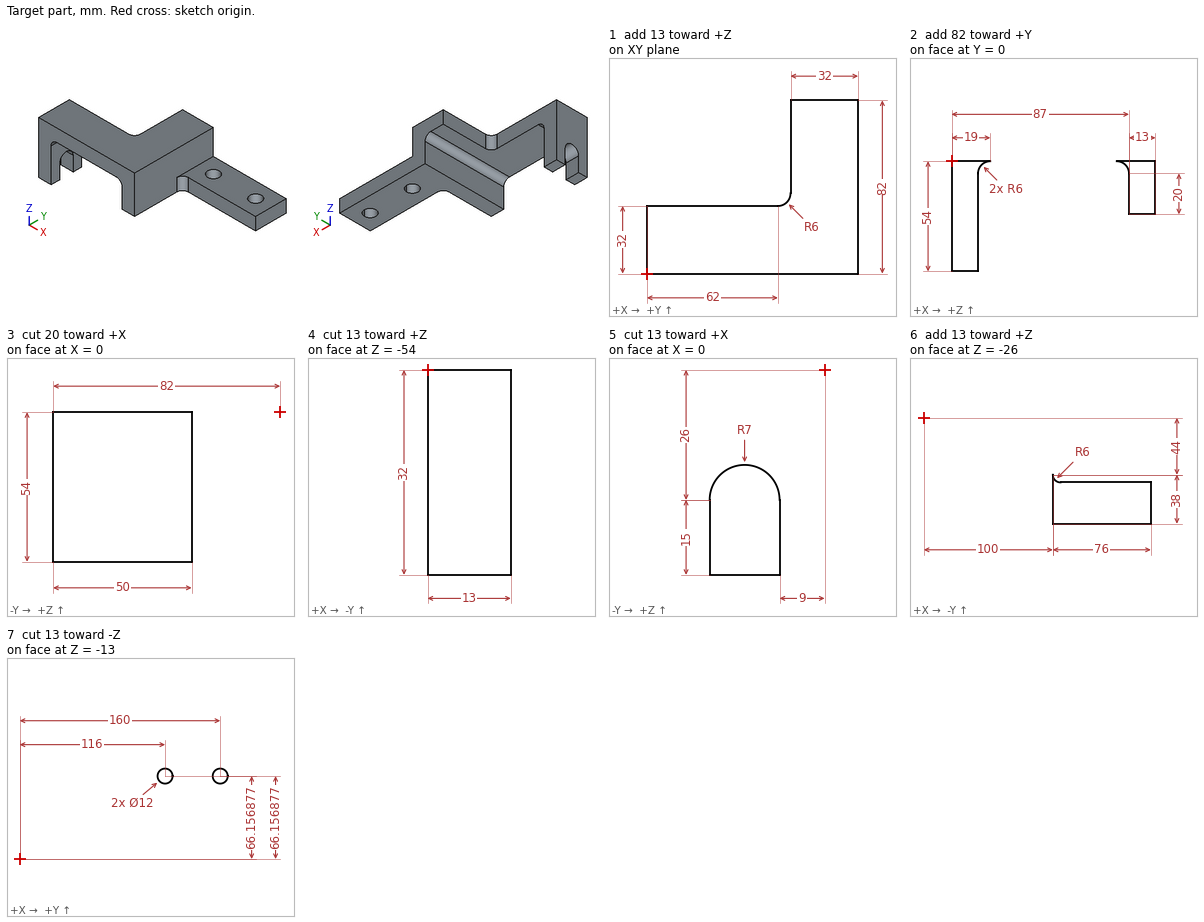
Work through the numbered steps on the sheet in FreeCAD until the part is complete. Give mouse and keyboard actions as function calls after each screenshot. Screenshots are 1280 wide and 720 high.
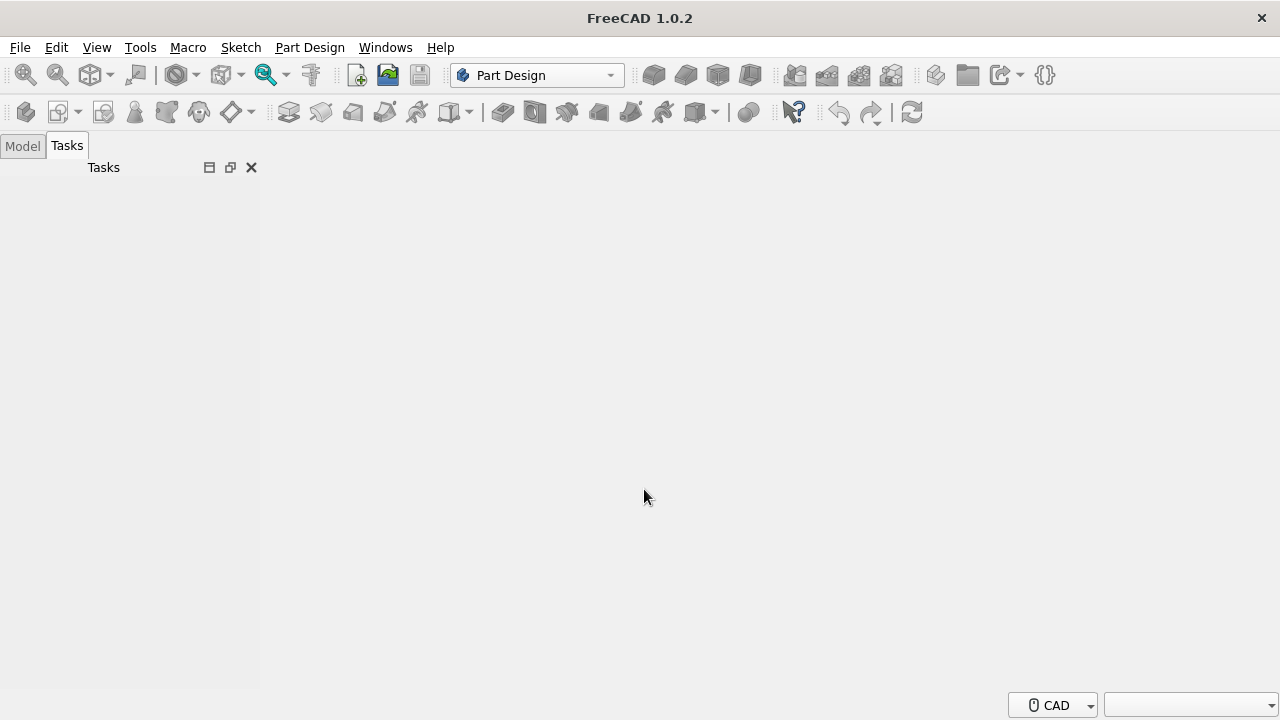
click(356, 76)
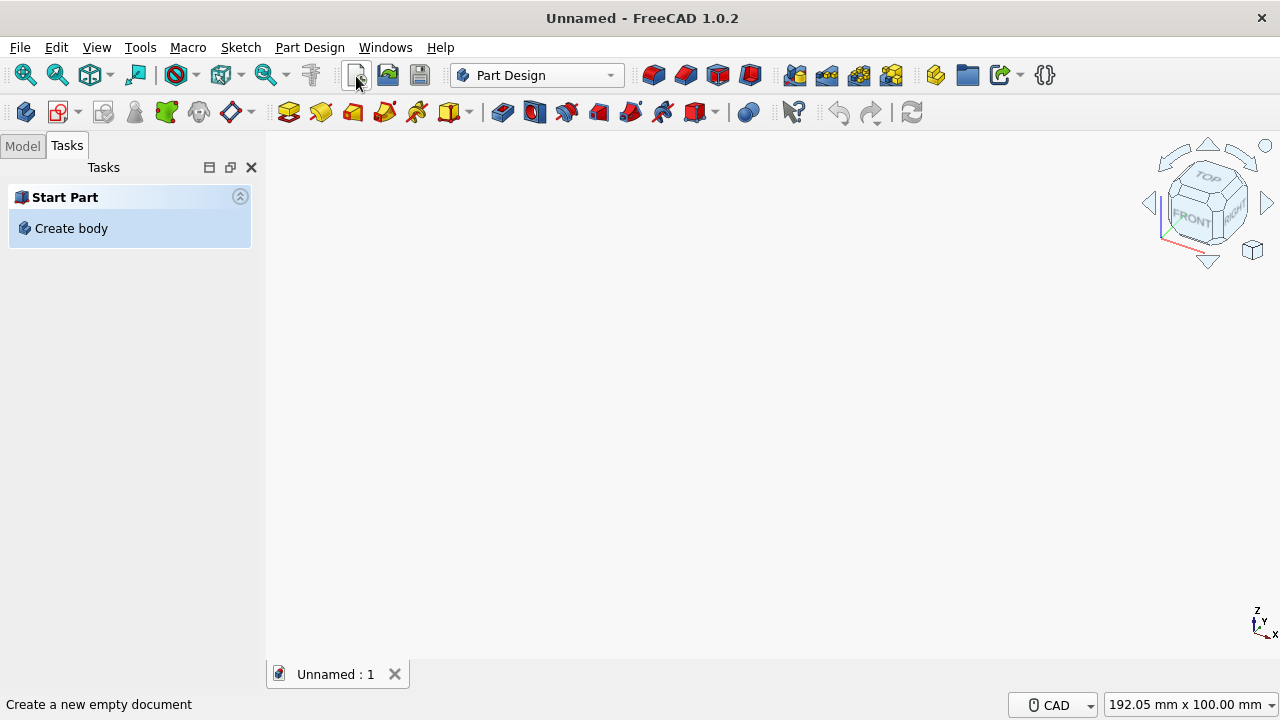
click(58, 112)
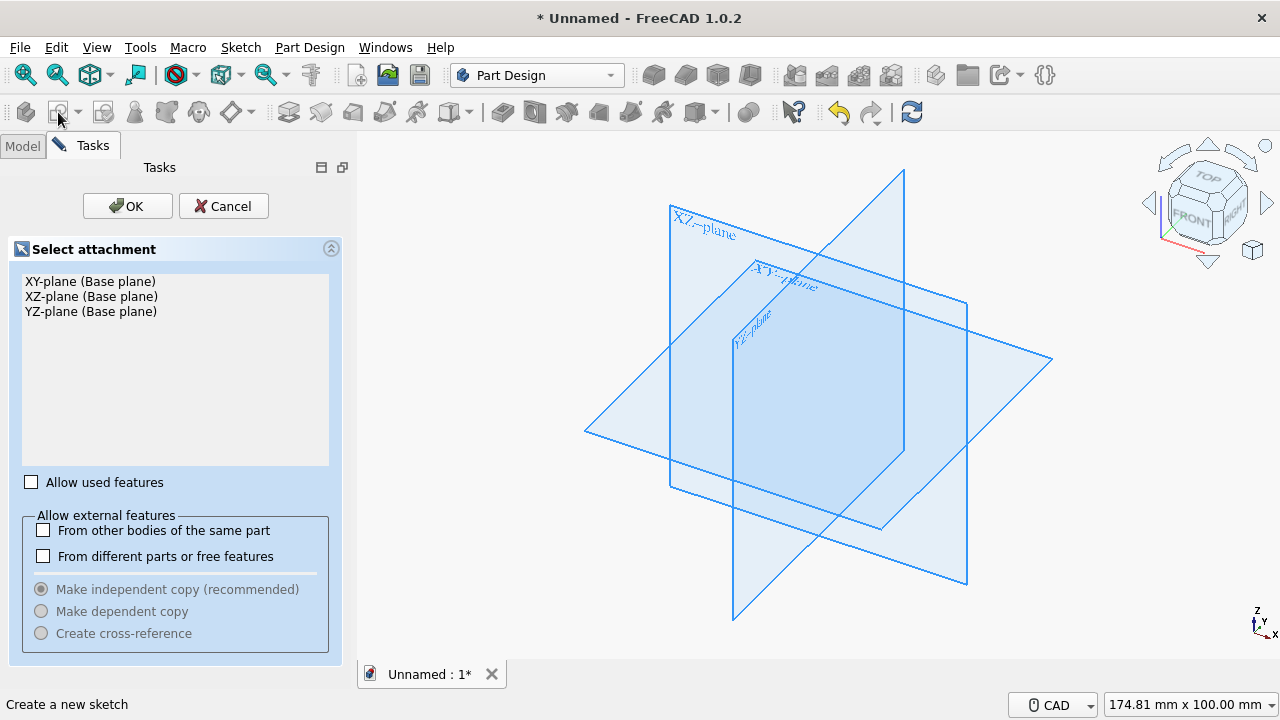
click(82, 282)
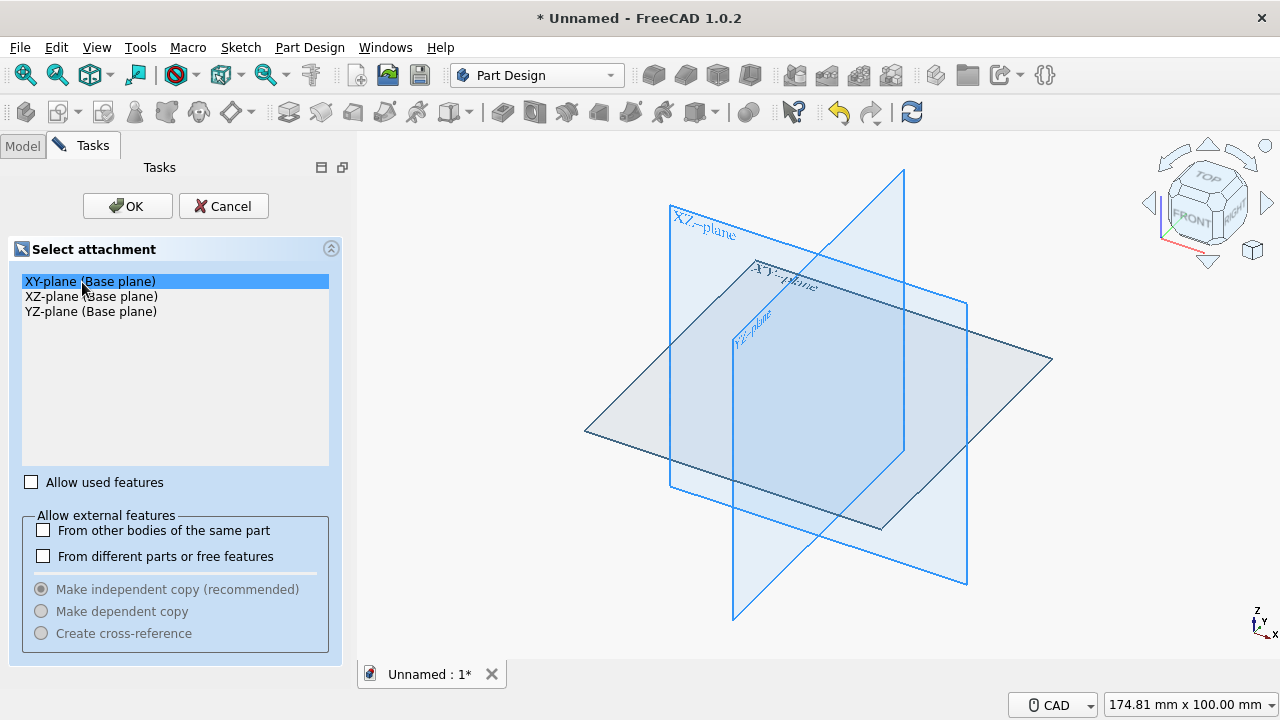
click(128, 206)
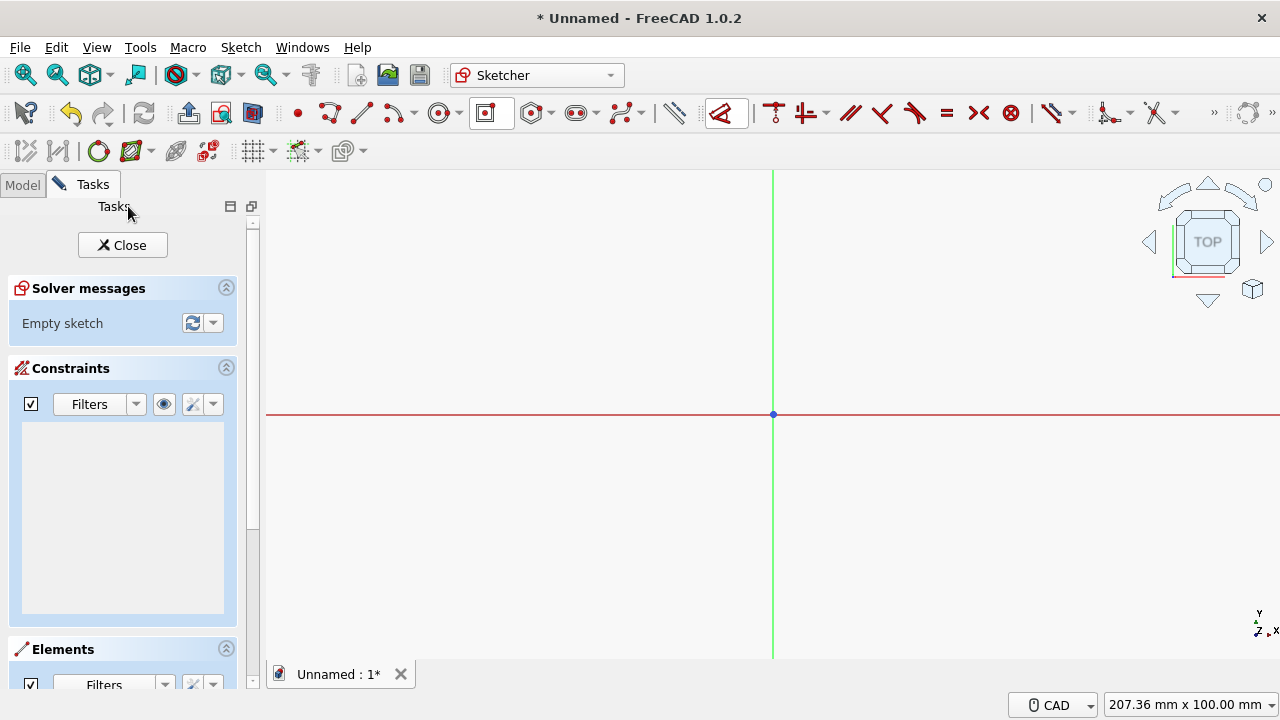
scroll(324, 631, down, 3)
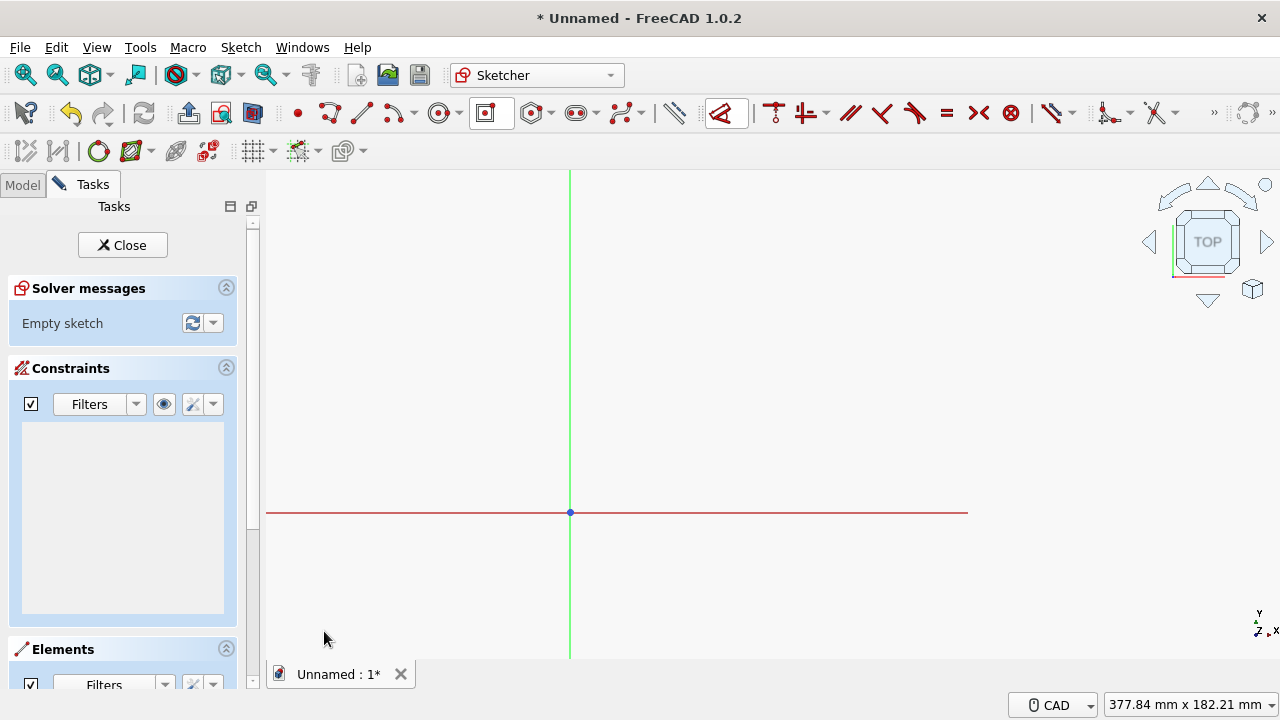
scroll(705, 378, up, 2)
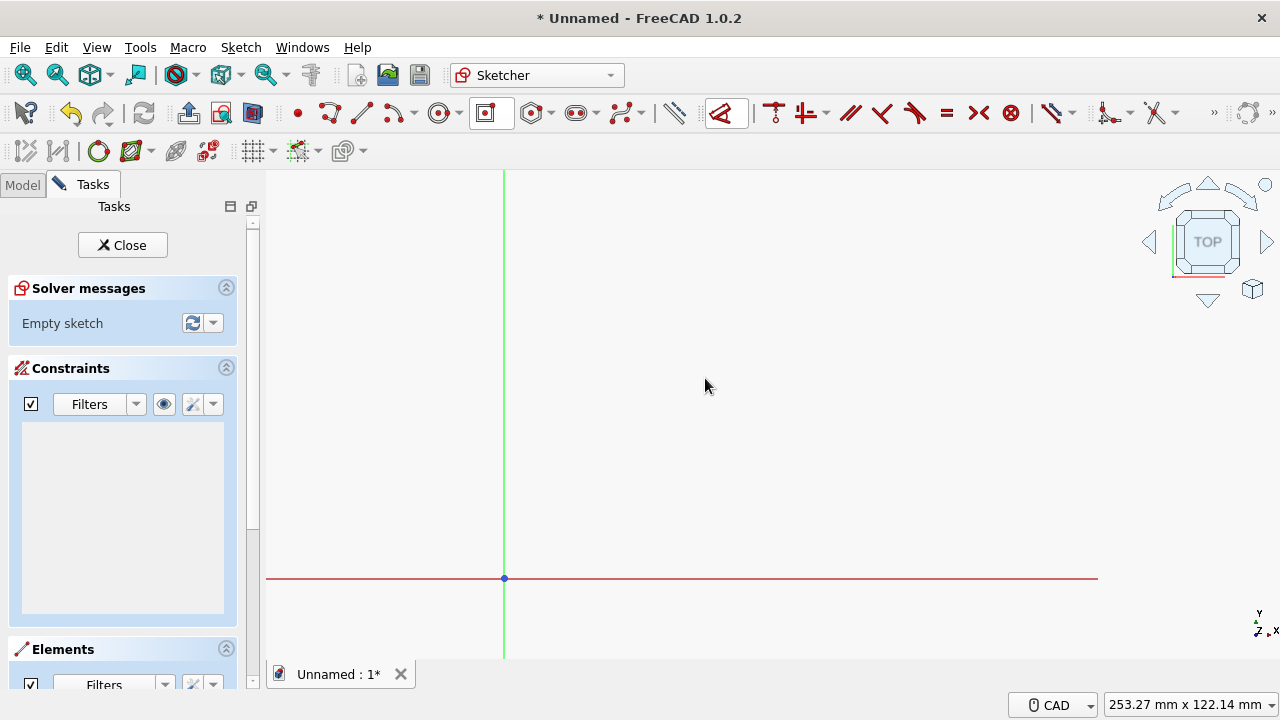
click(330, 114)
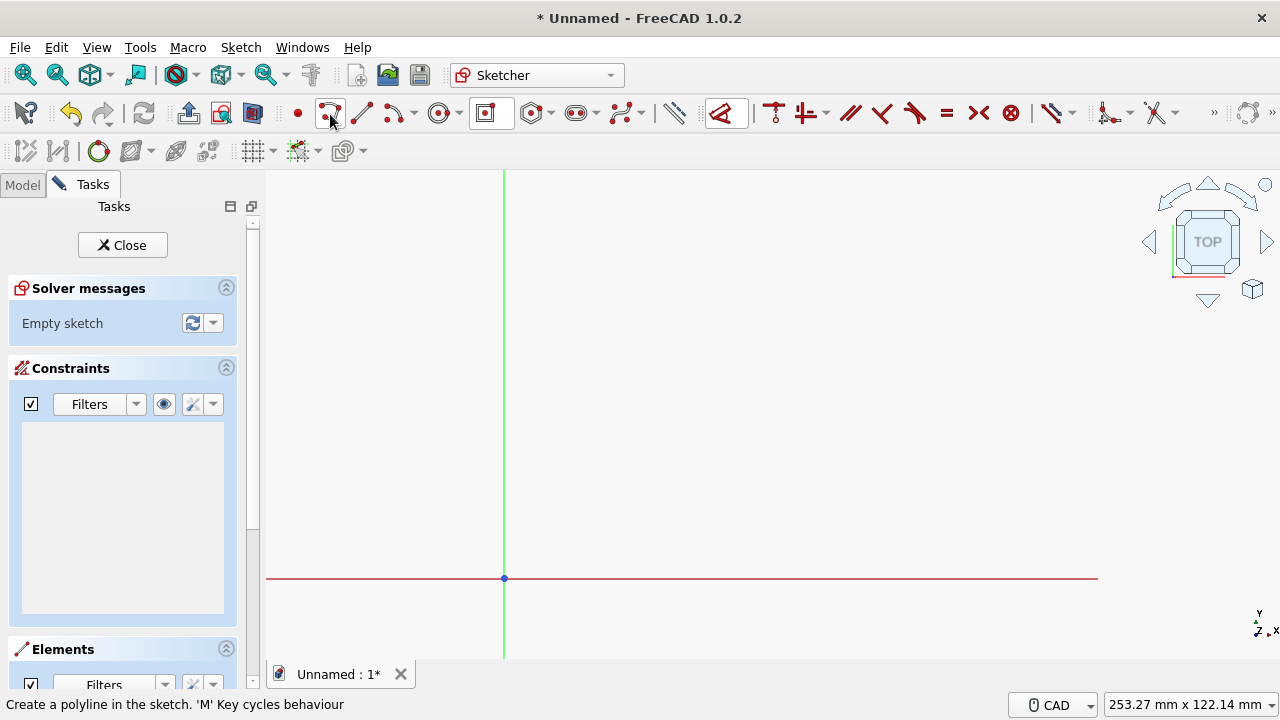
click(752, 450)
click(504, 450)
click(504, 579)
click(904, 570)
click(904, 250)
click(776, 250)
click(776, 426)
right_click(776, 426)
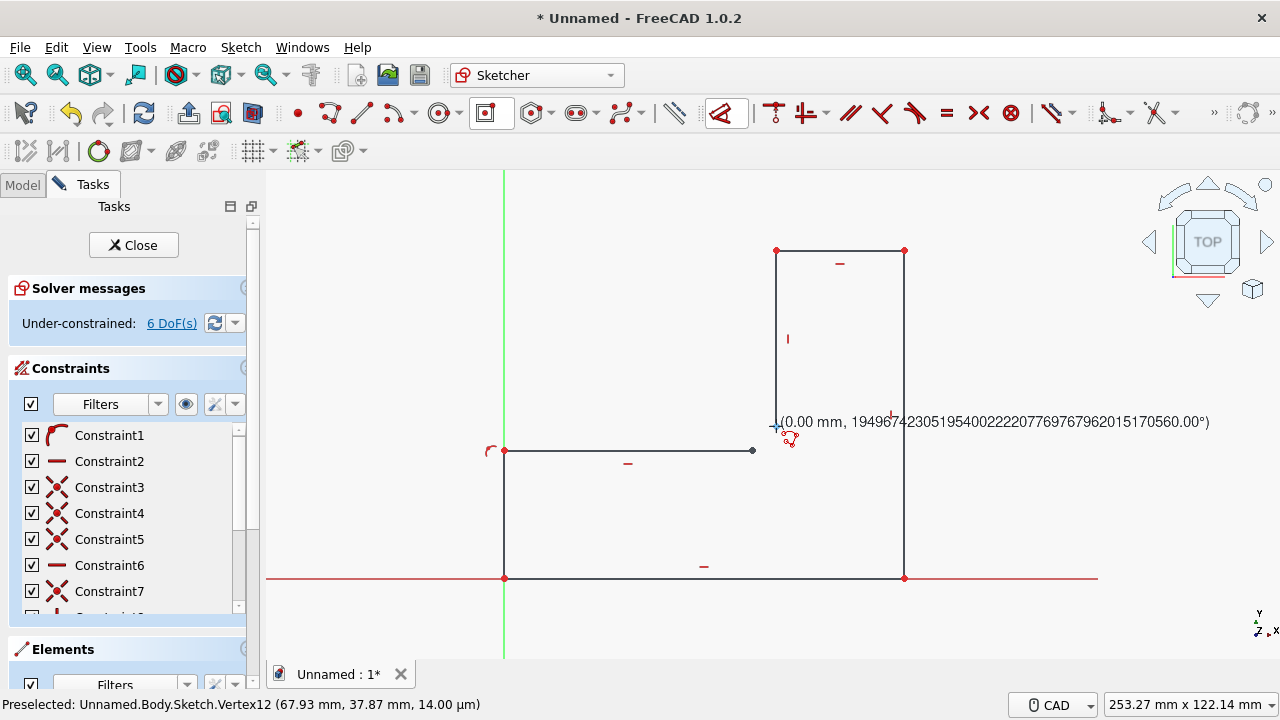
click(416, 114)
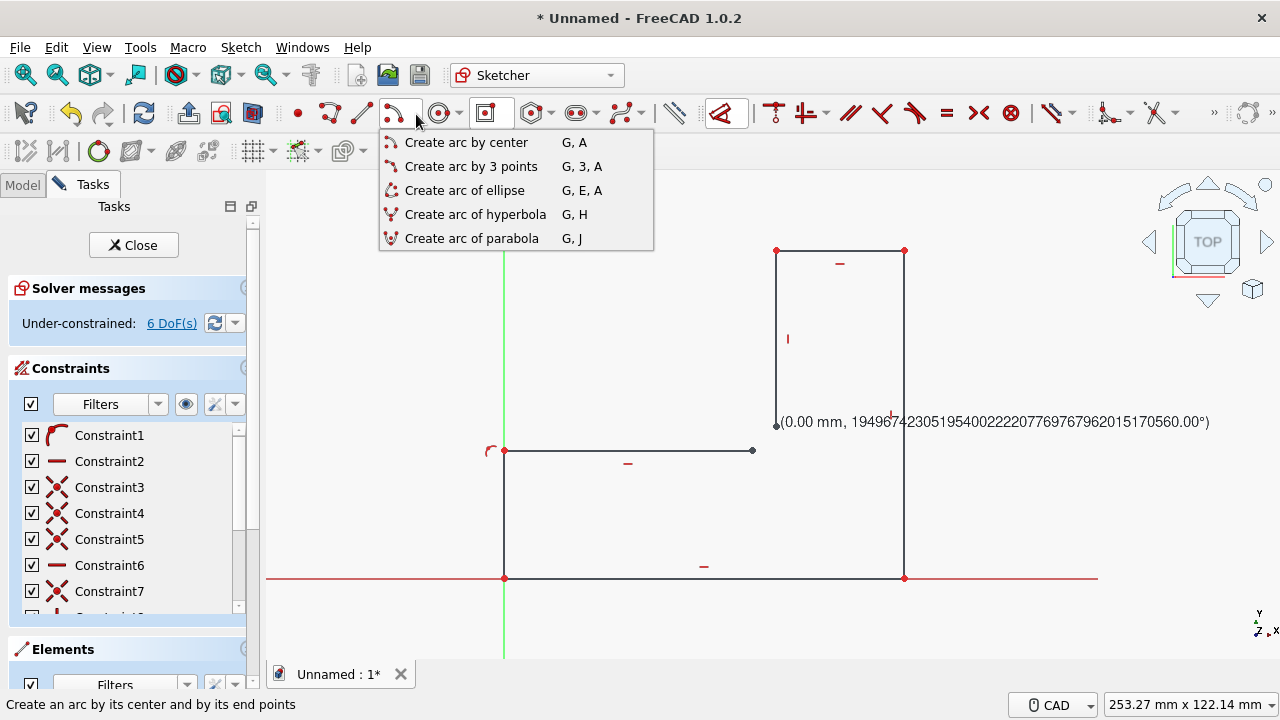
click(516, 166)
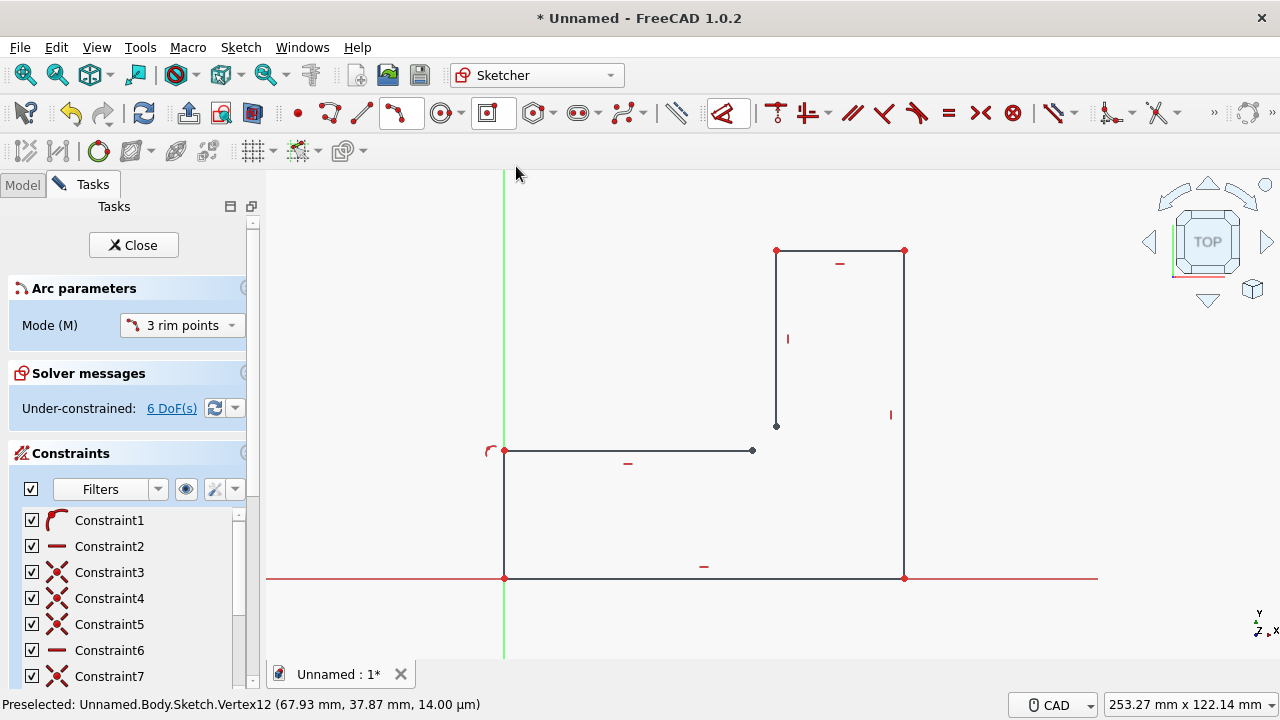
click(776, 427)
click(752, 451)